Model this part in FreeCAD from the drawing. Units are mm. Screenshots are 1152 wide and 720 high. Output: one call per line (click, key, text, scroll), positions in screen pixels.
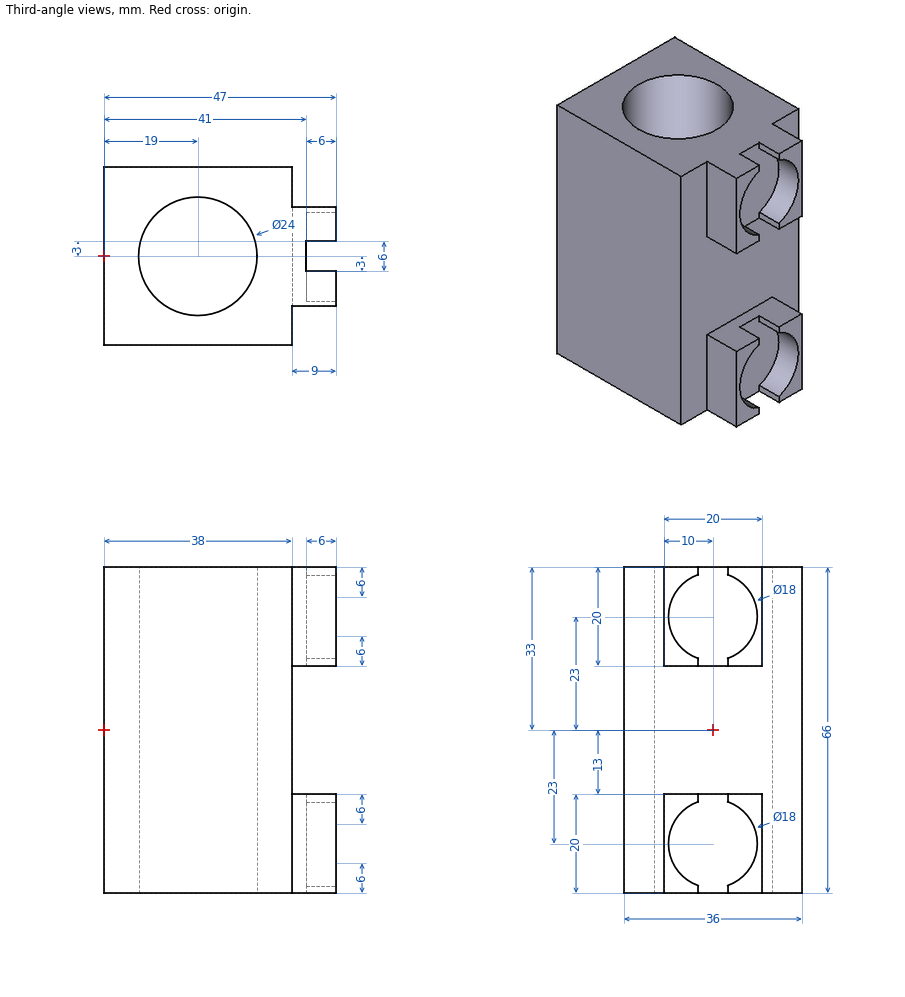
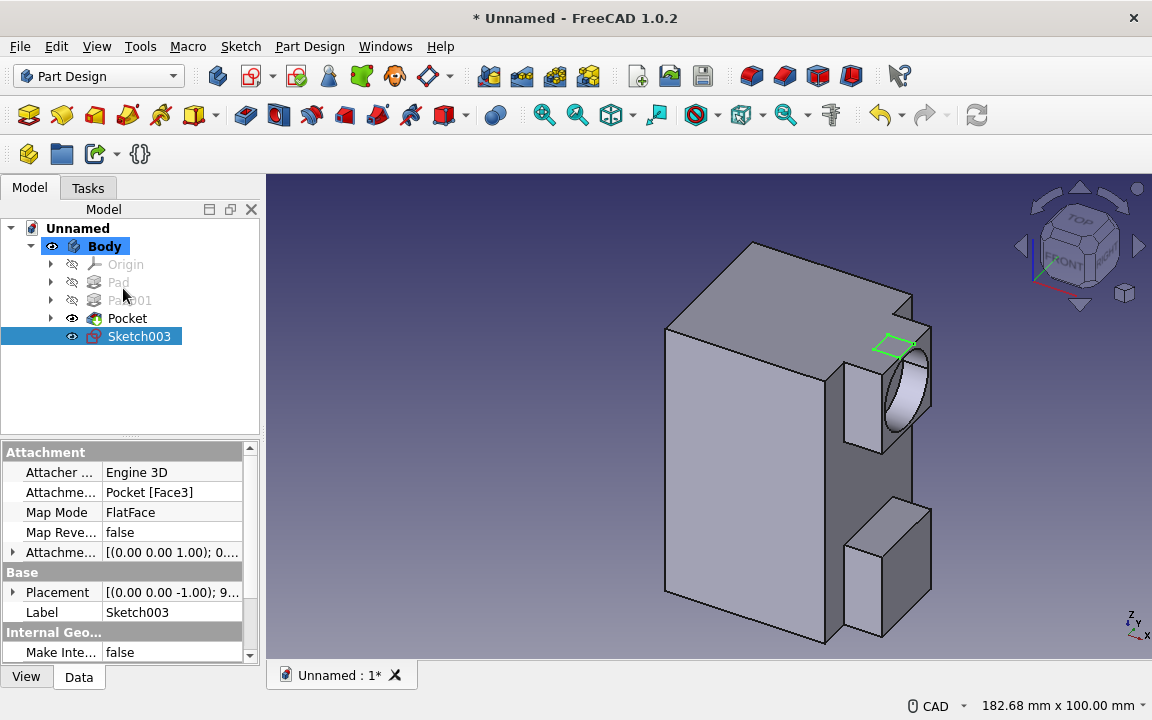
click(246, 116)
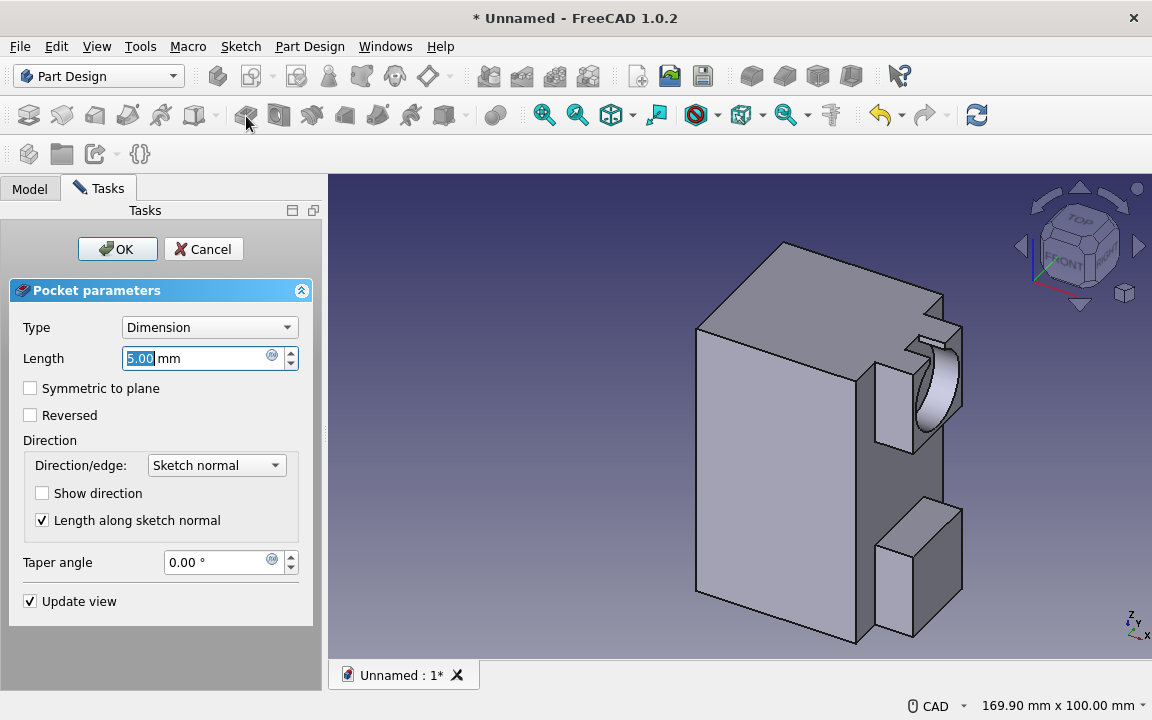
click(210, 328)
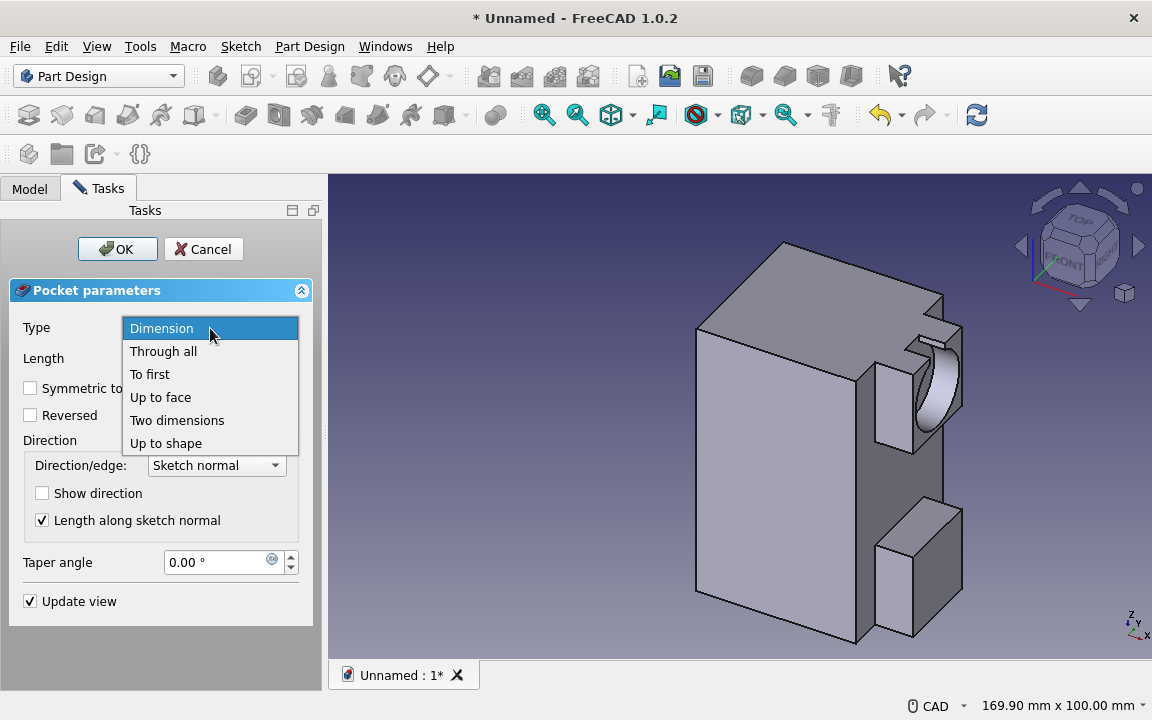
click(208, 420)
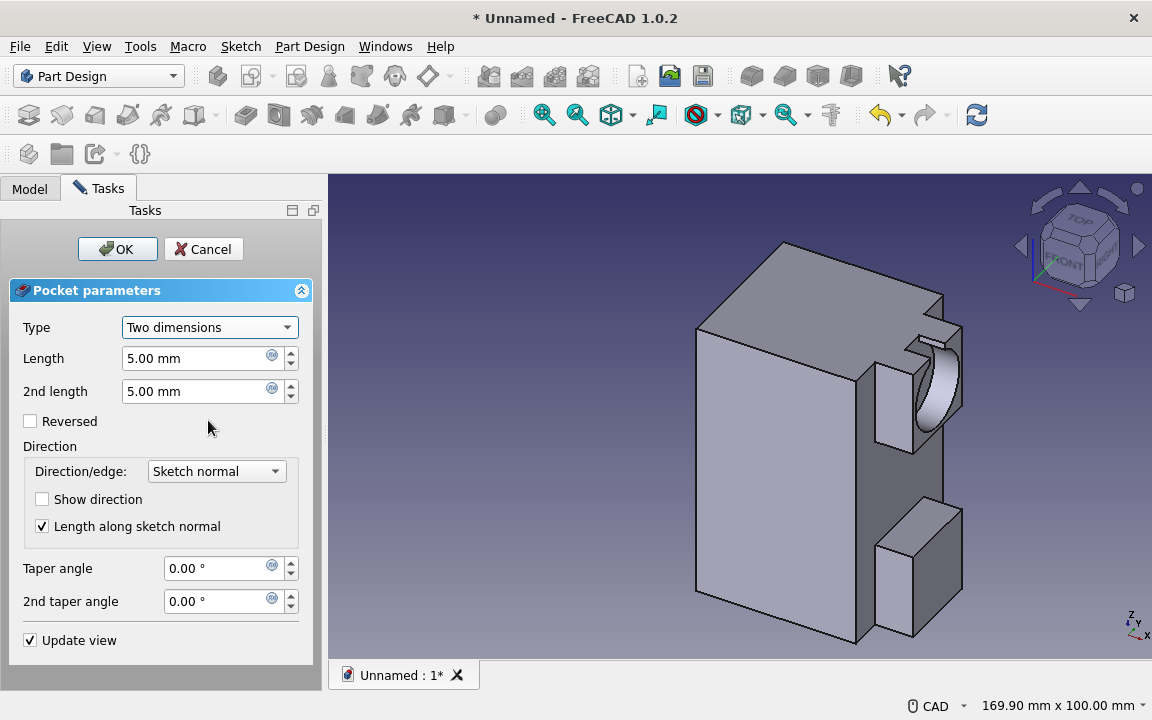
triple_click(204, 358)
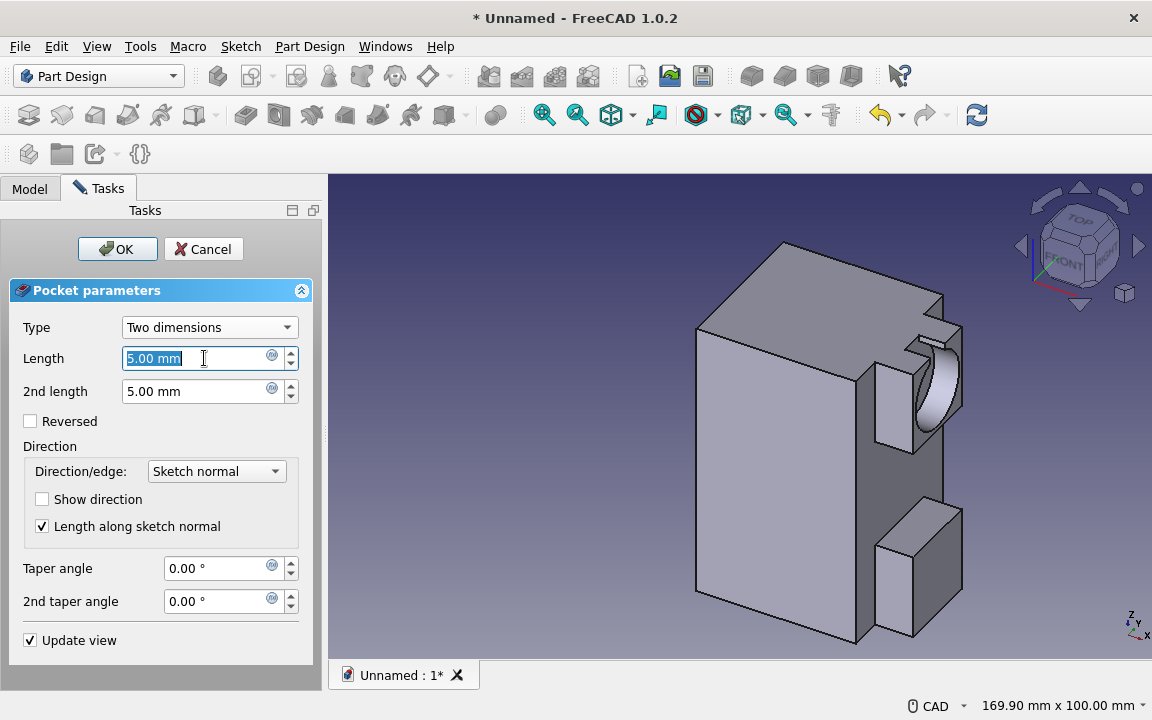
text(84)
key(Tab)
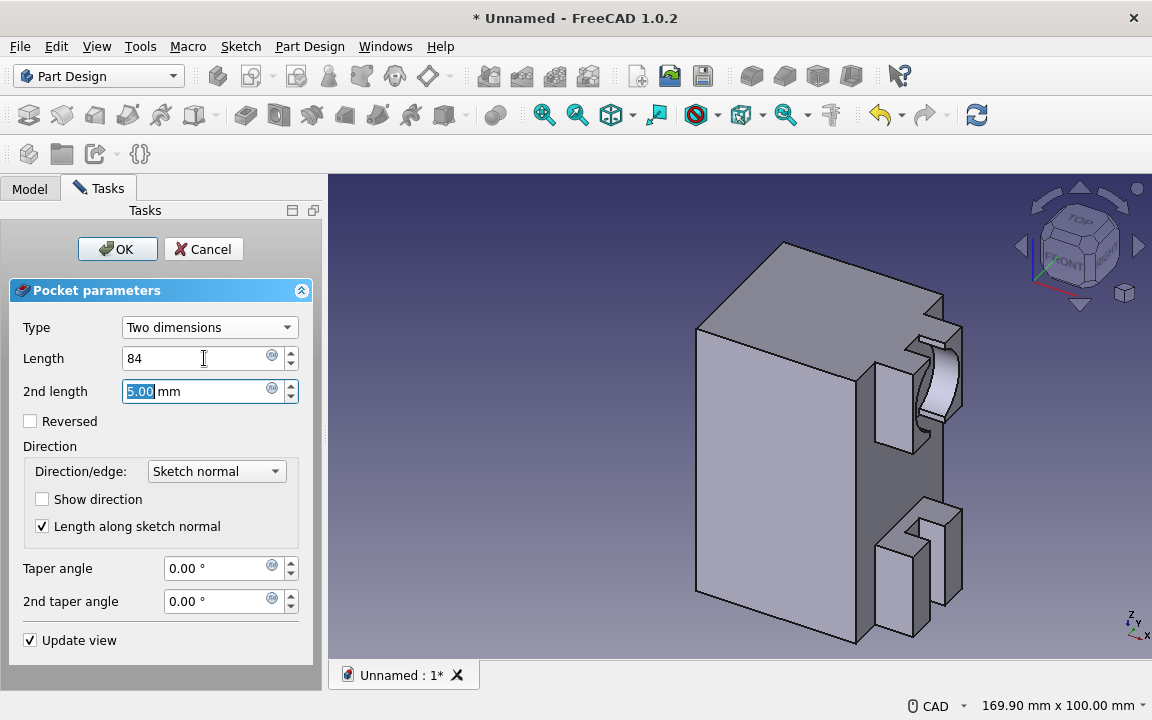
text(6)
key(Tab)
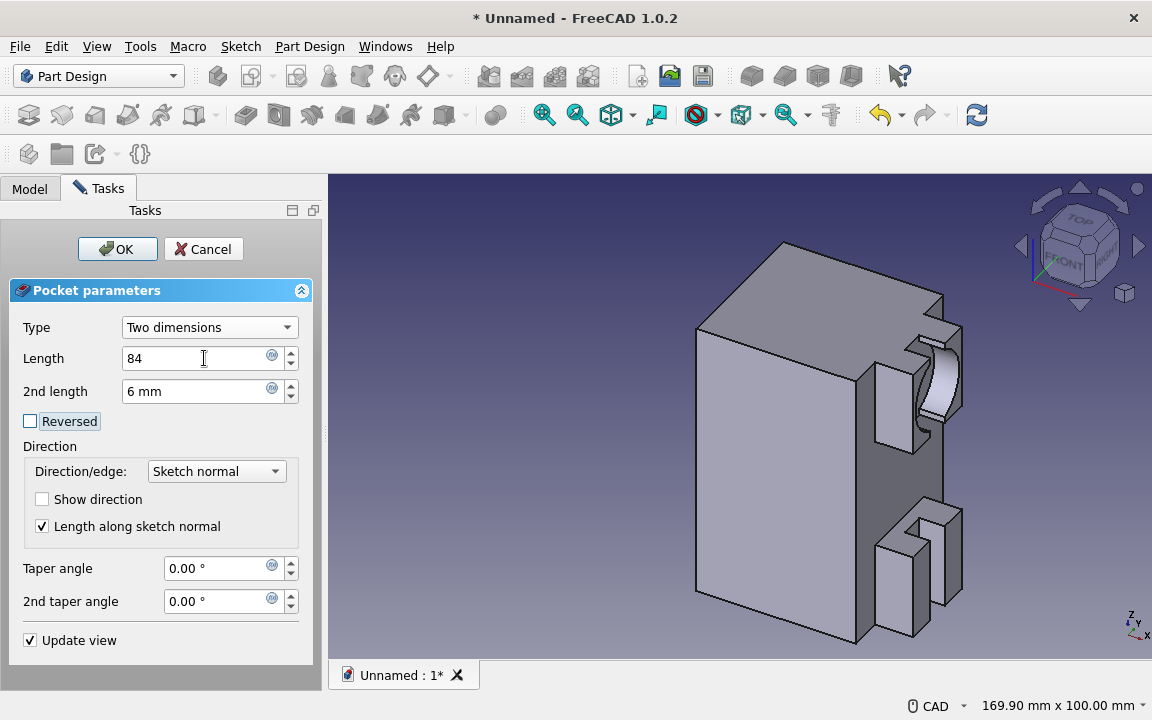
click(31, 421)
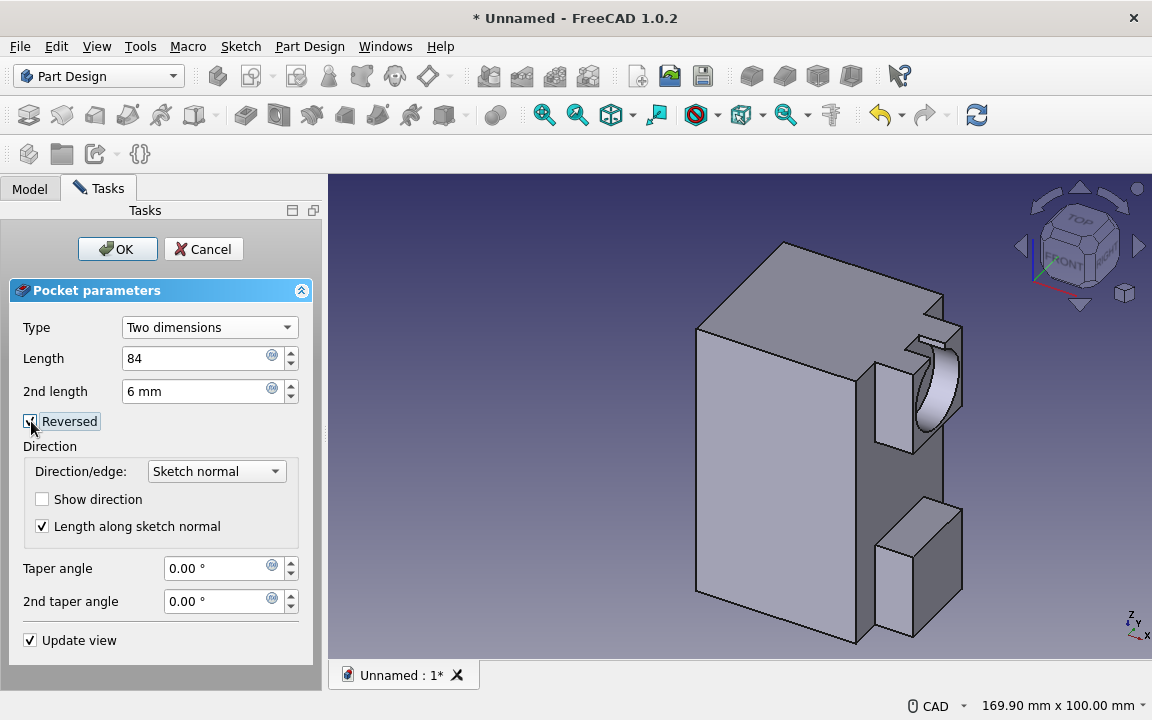
click(118, 249)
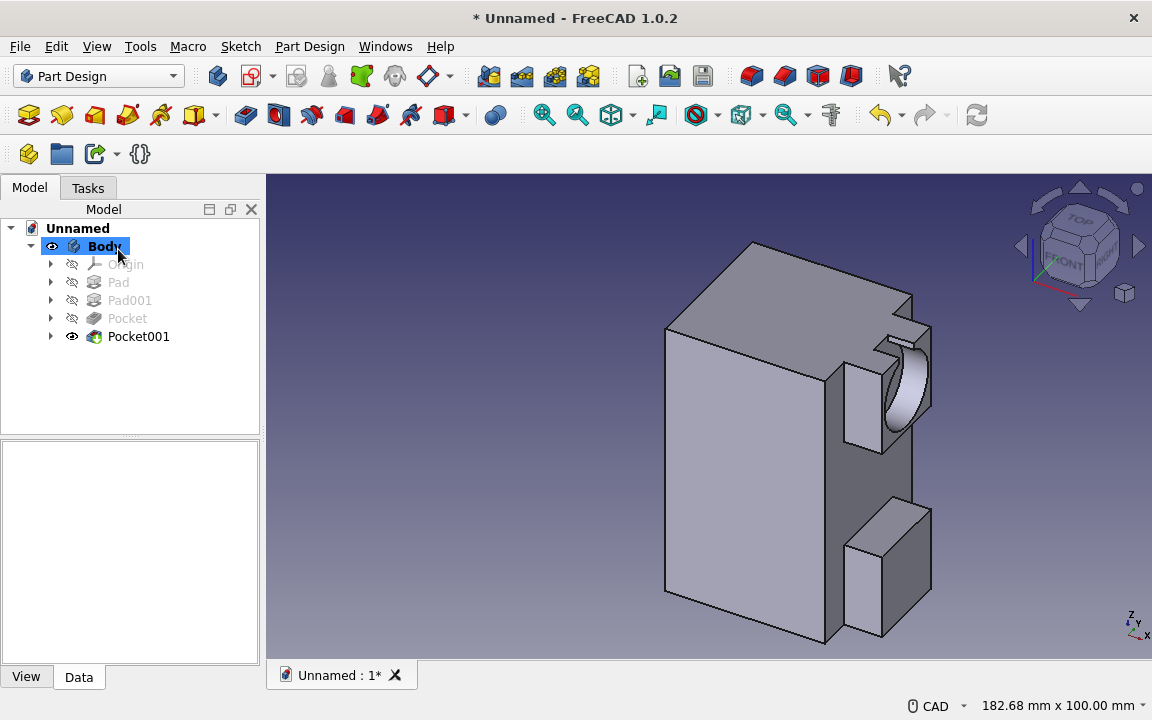
click(51, 264)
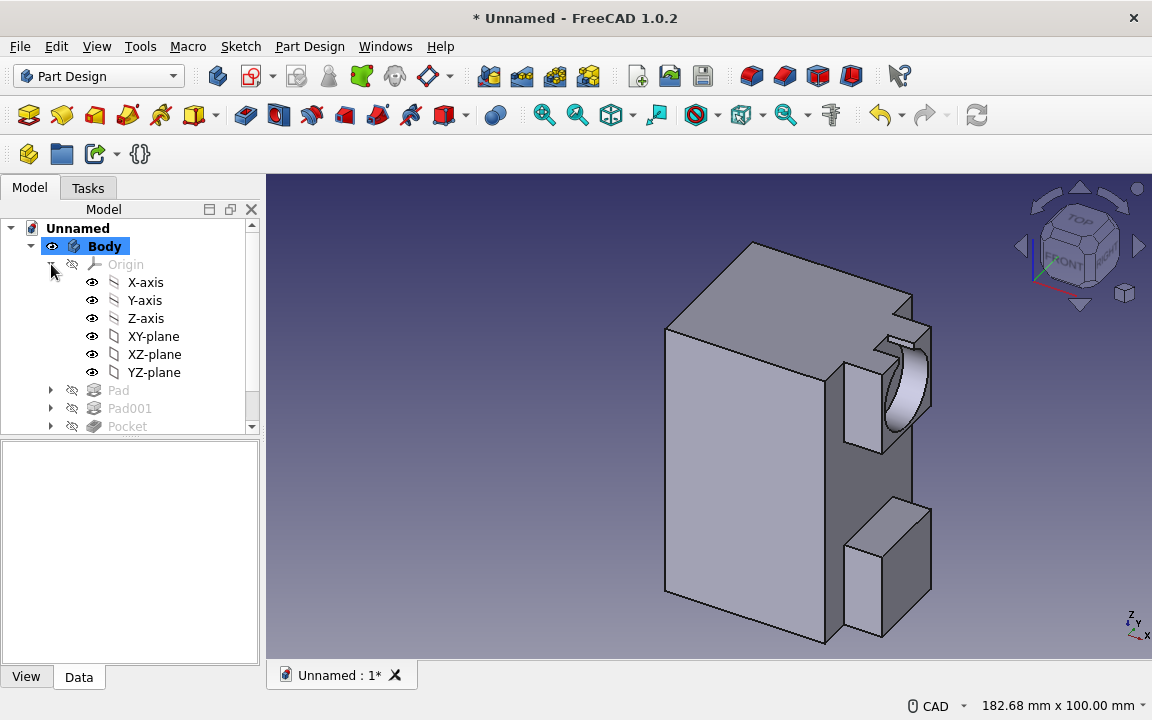
click(137, 336)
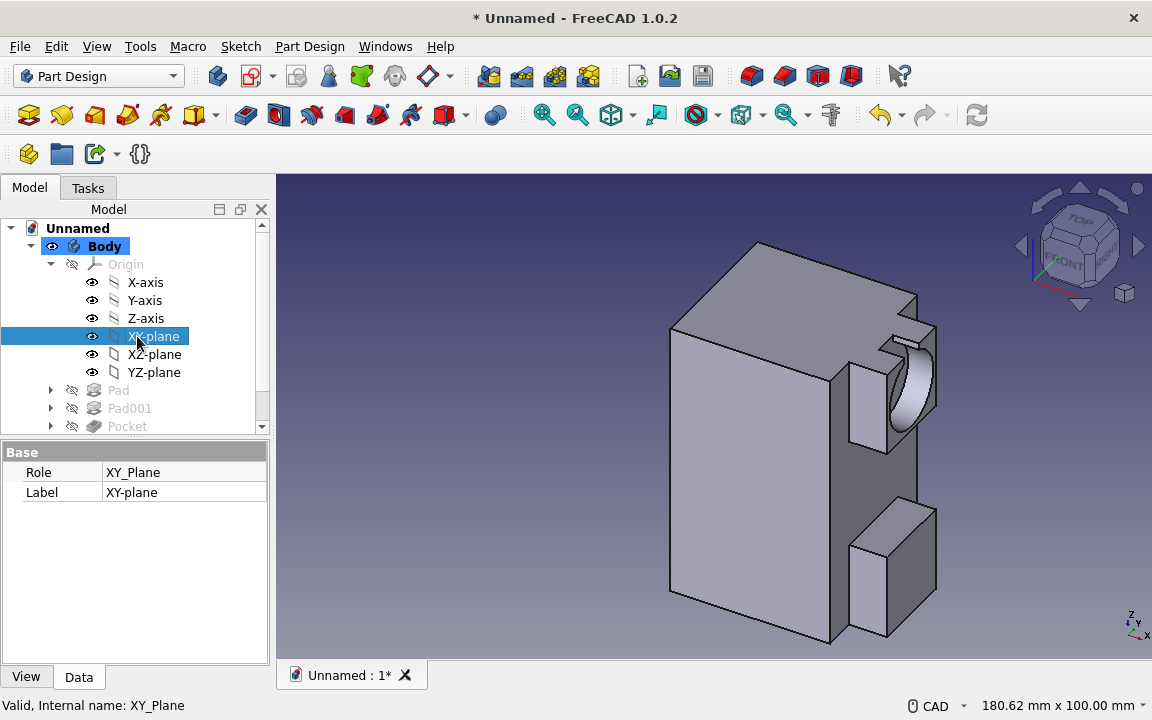
click(428, 76)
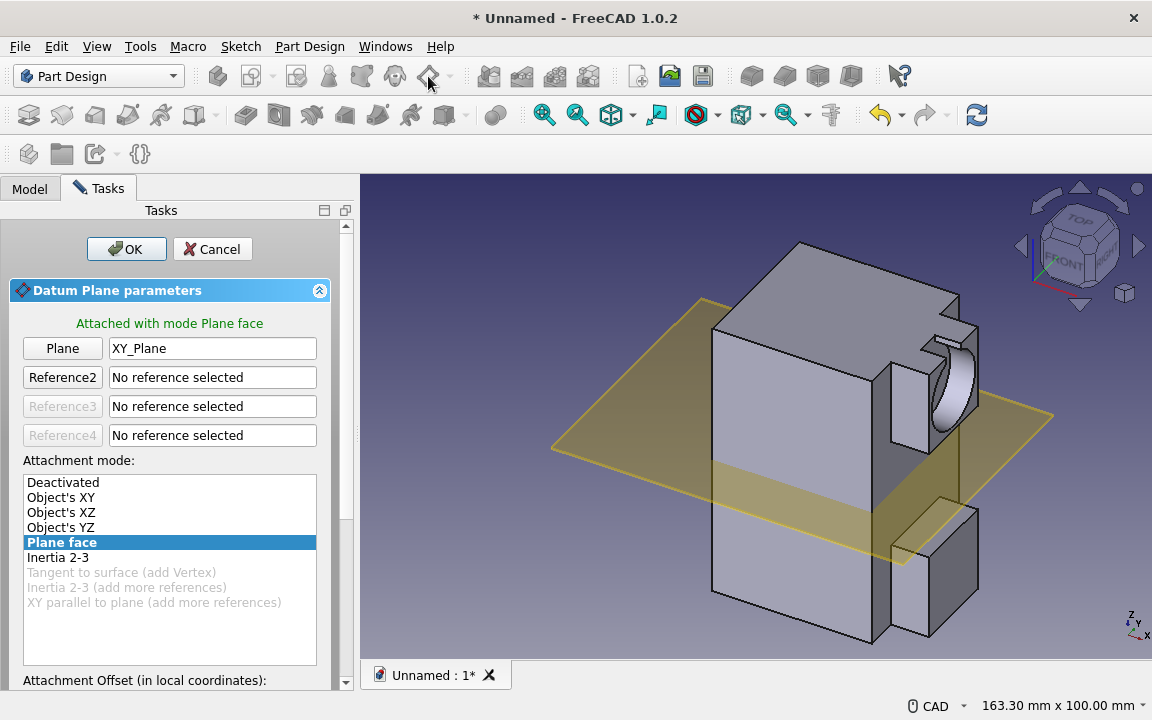
scroll(346, 455, down, 3)